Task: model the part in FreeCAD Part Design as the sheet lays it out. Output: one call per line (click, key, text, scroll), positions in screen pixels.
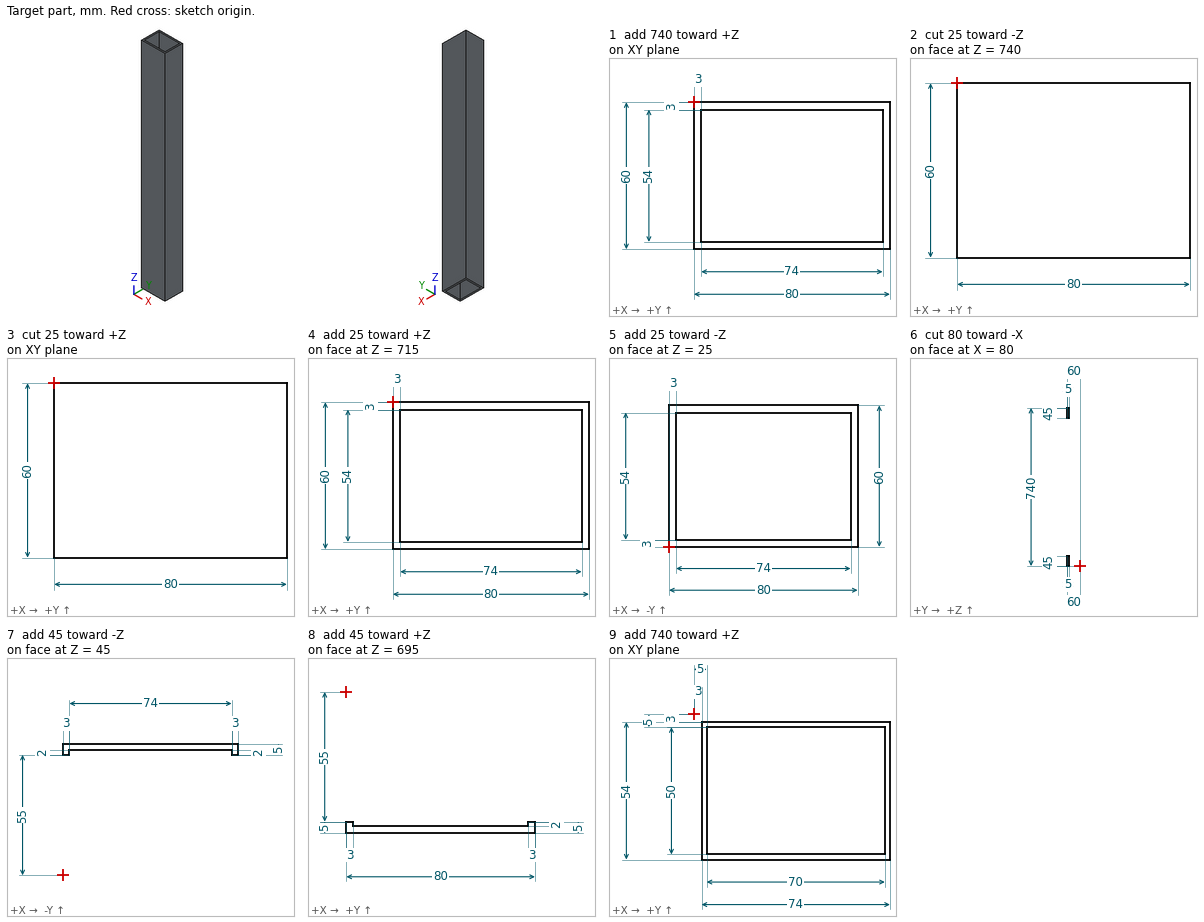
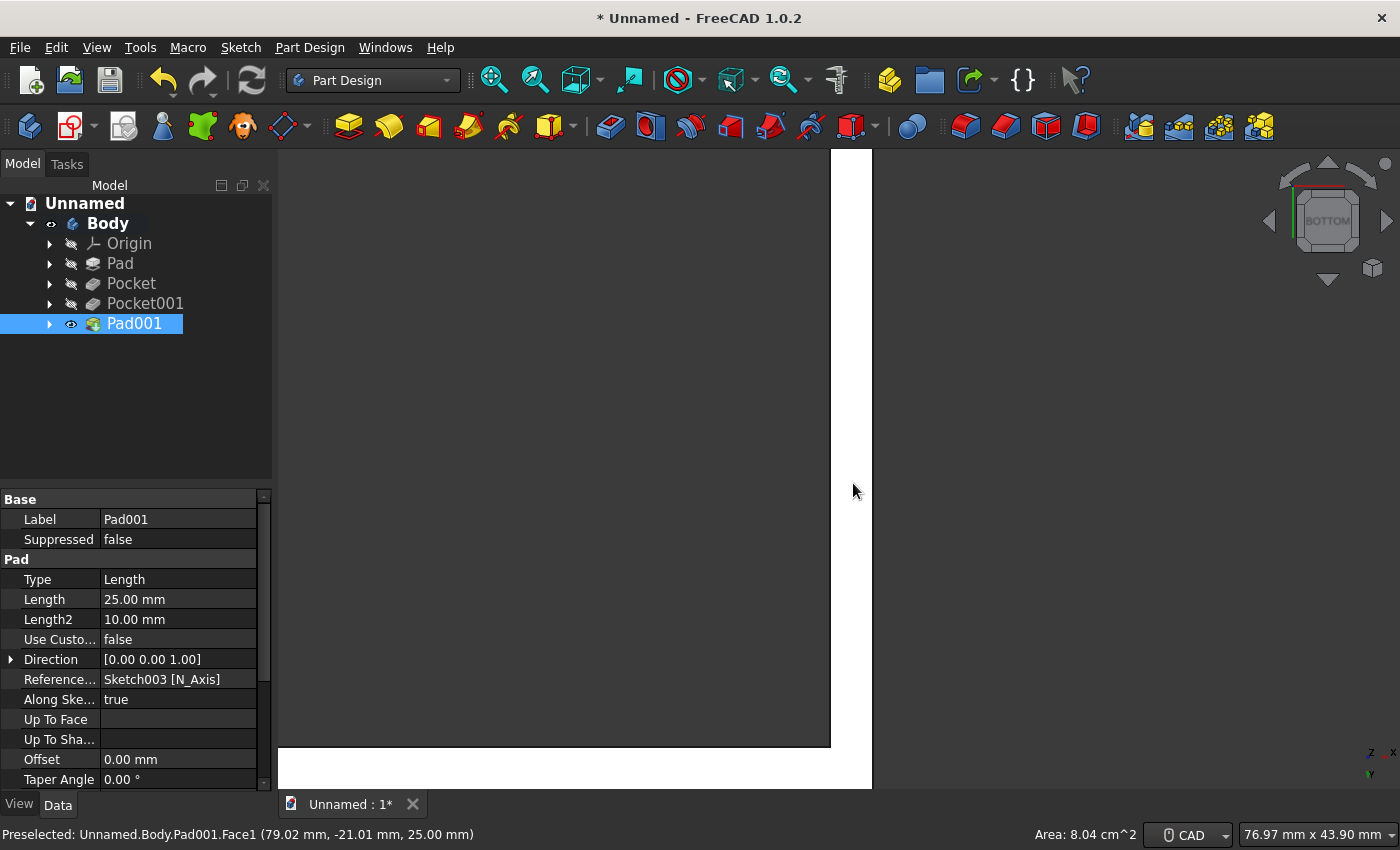
click(70, 126)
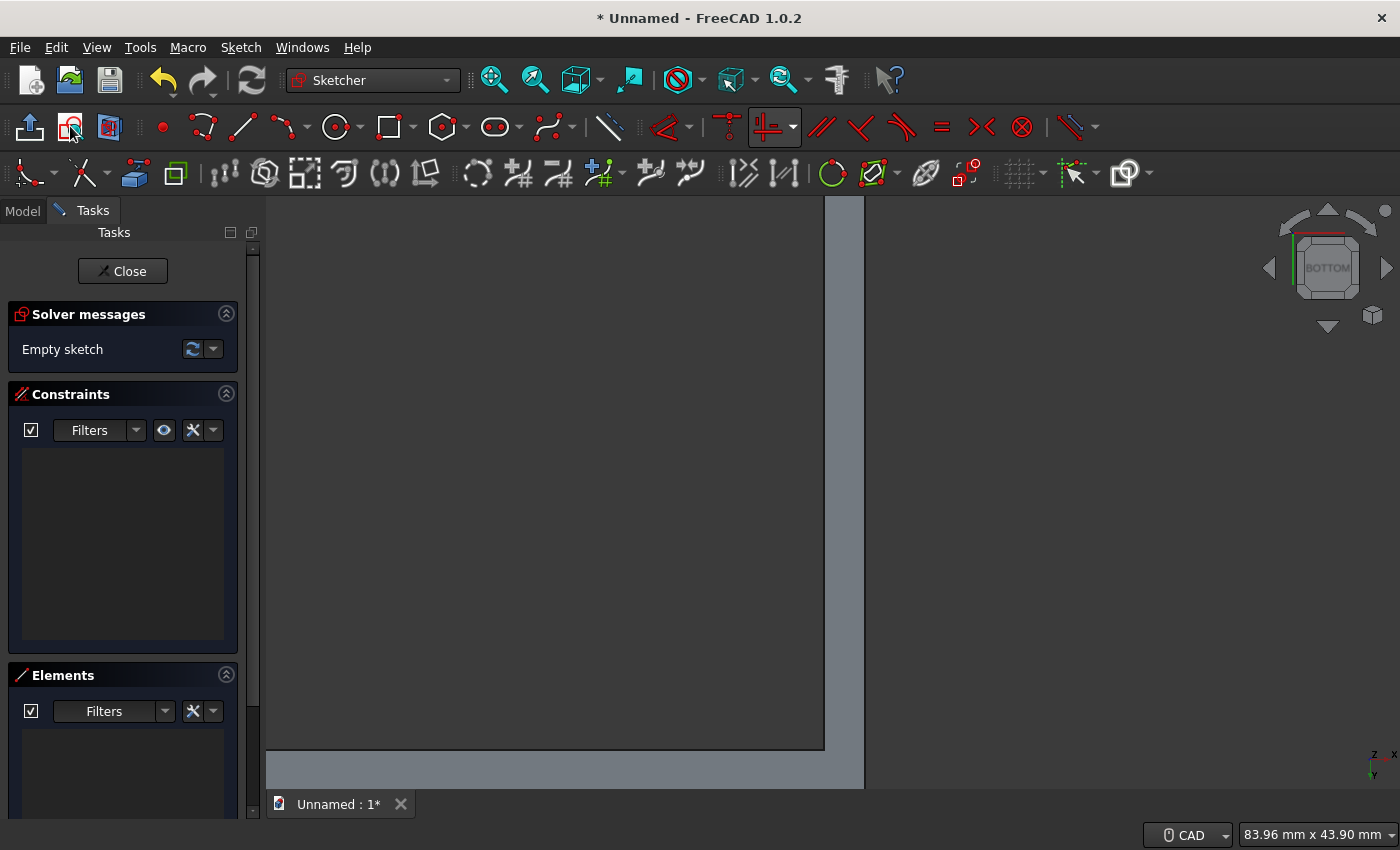
scroll(1123, 580, down, 4)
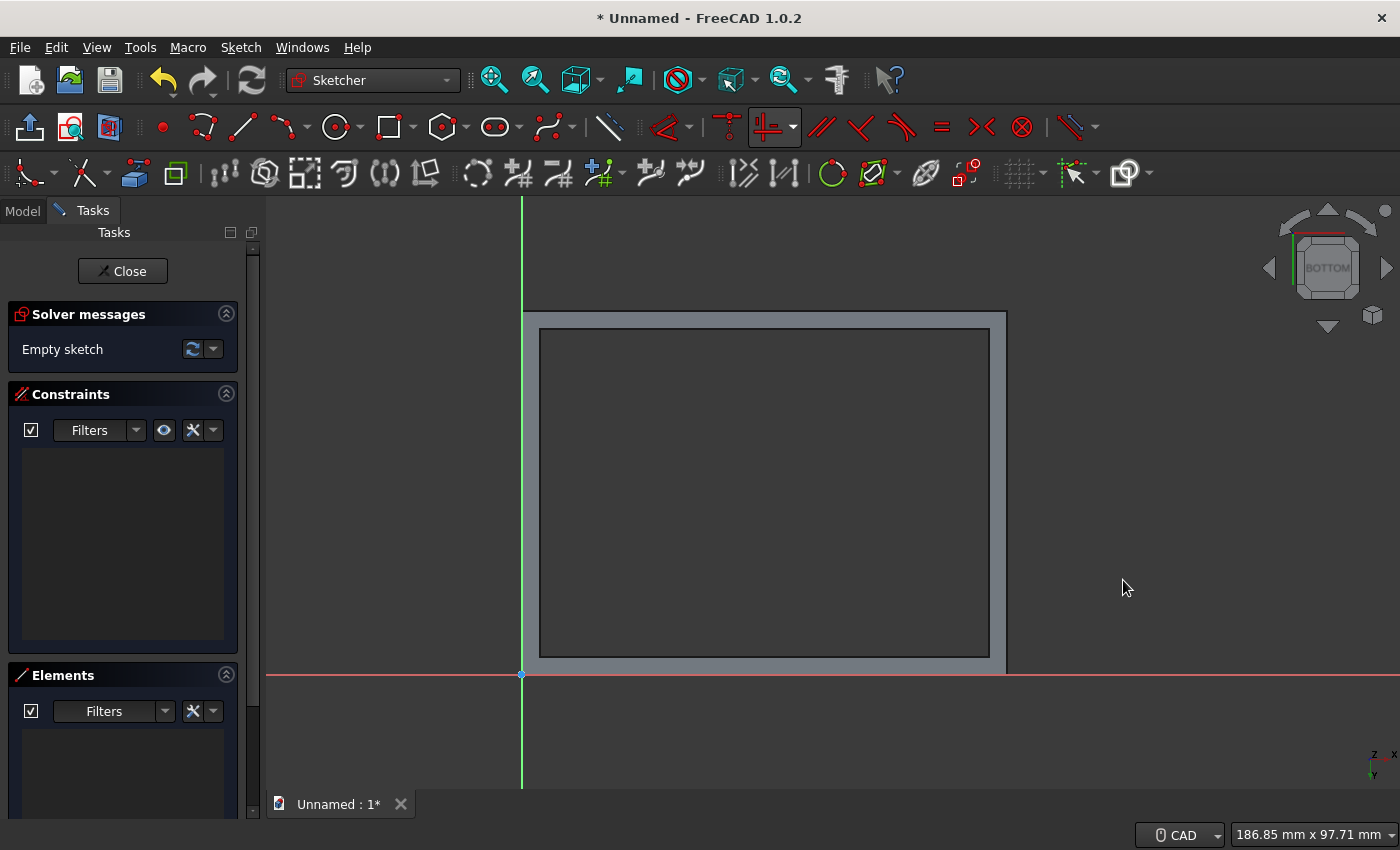
key(g)
key(r)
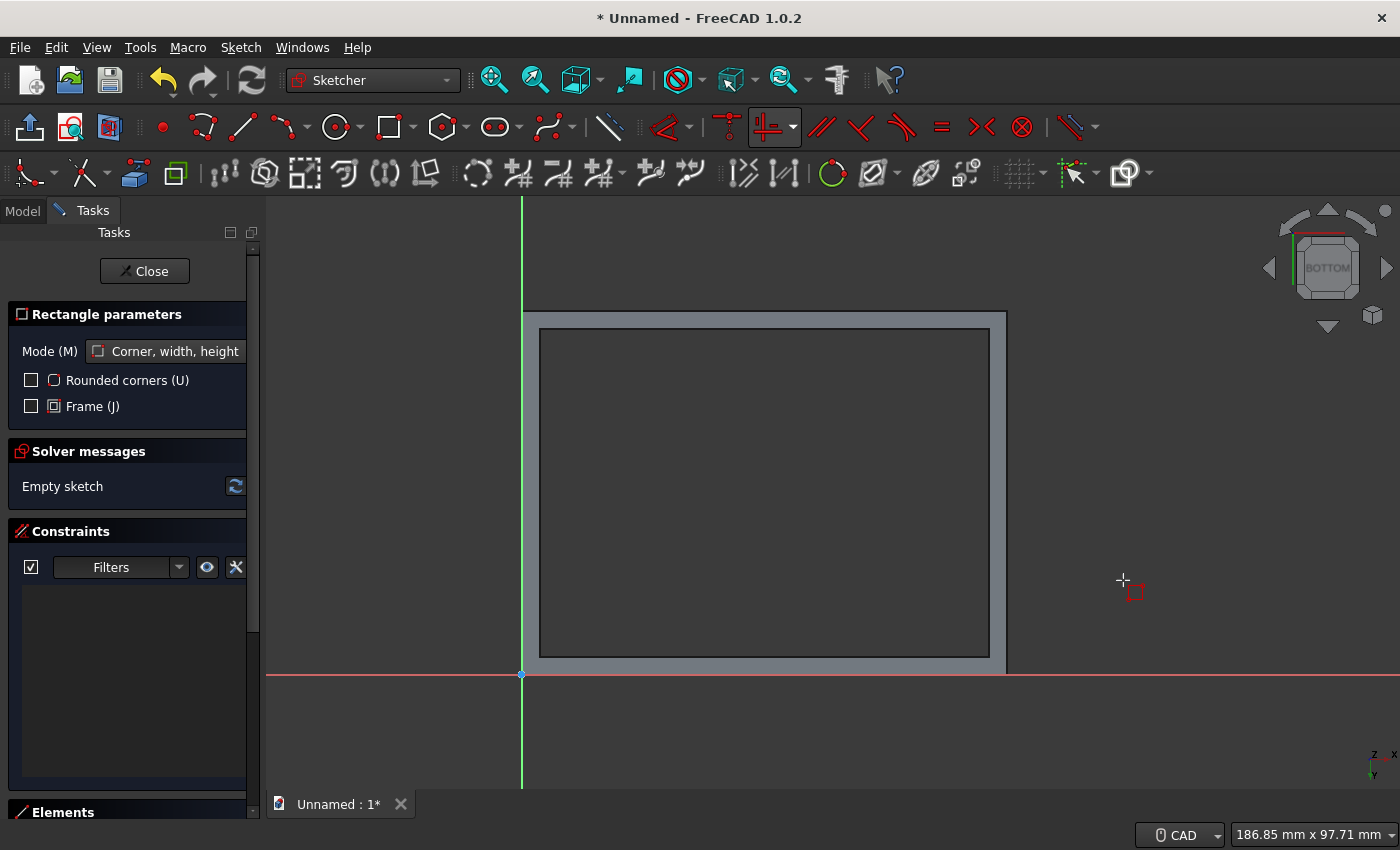
click(522, 675)
click(1007, 311)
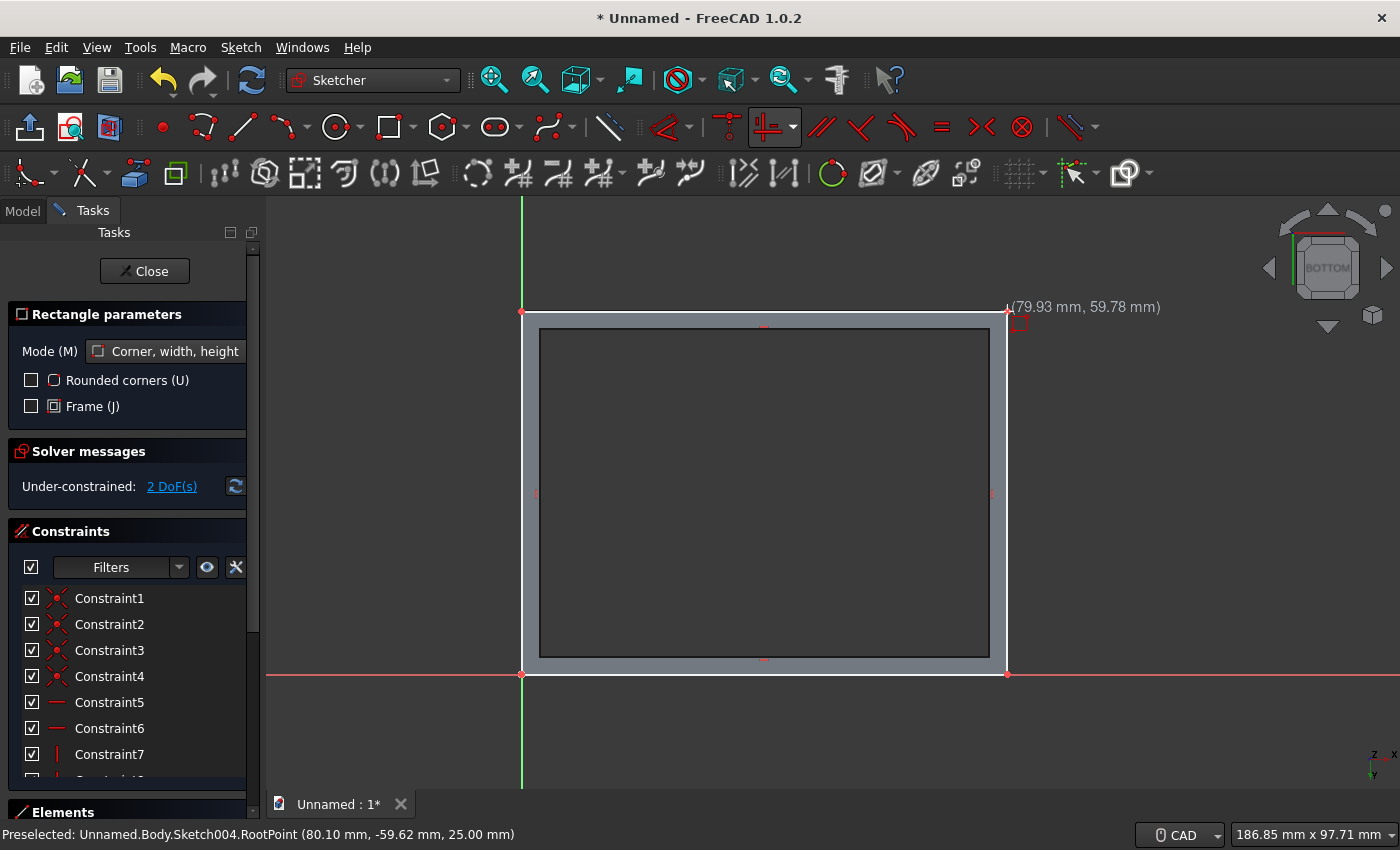
click(540, 329)
click(989, 657)
key(Escape)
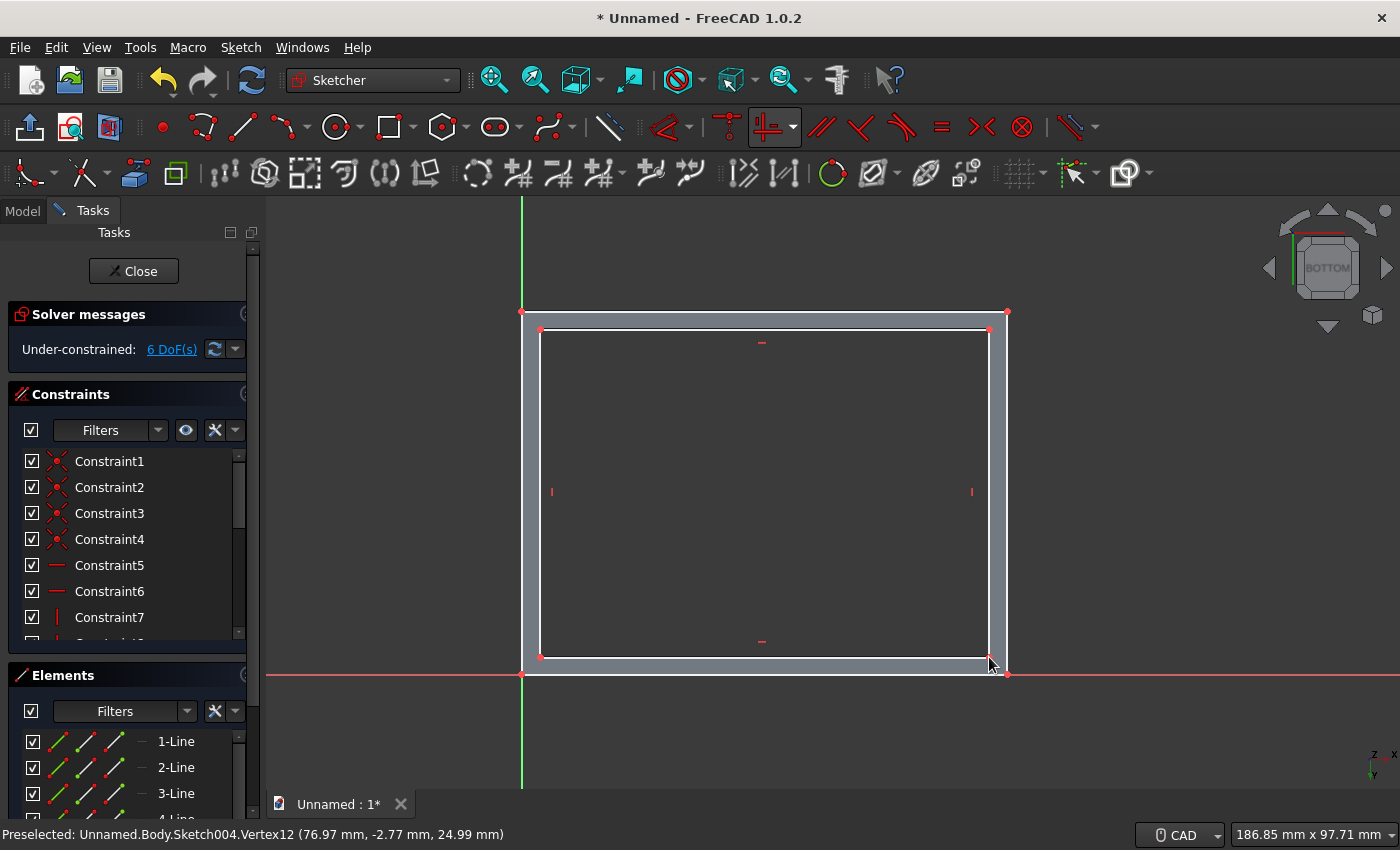
key(d)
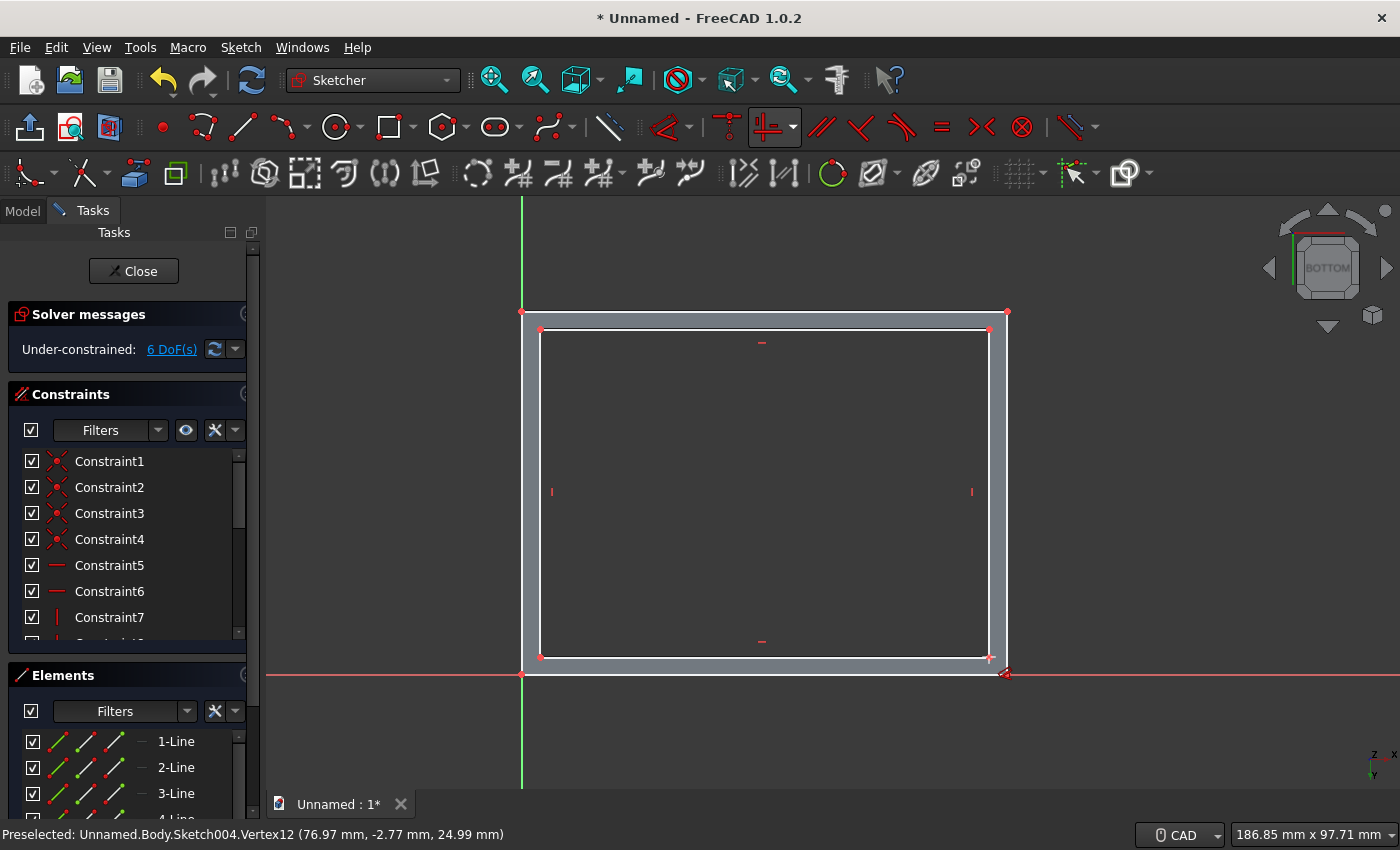
click(667, 675)
click(764, 709)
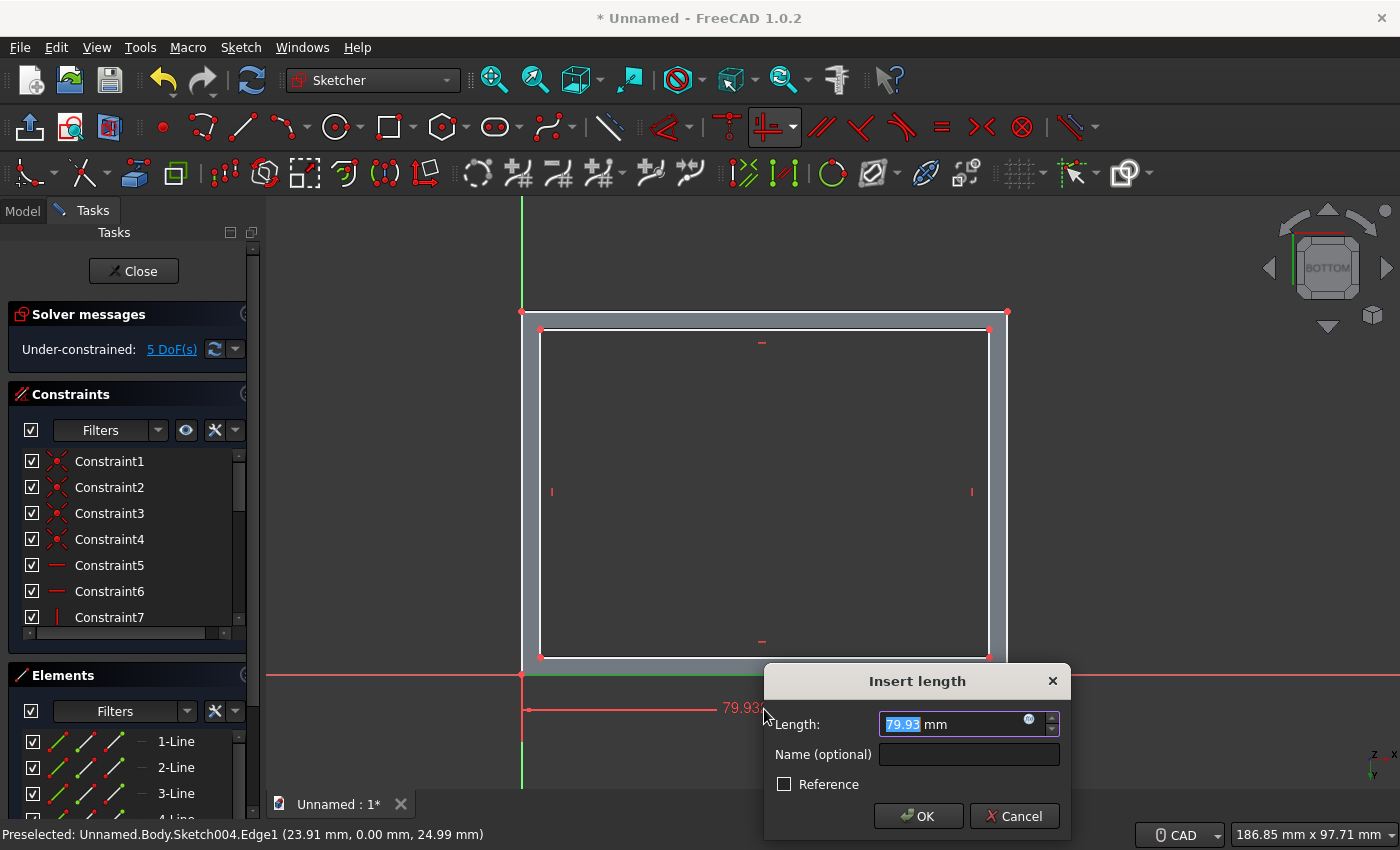
text(80)
key(Return)